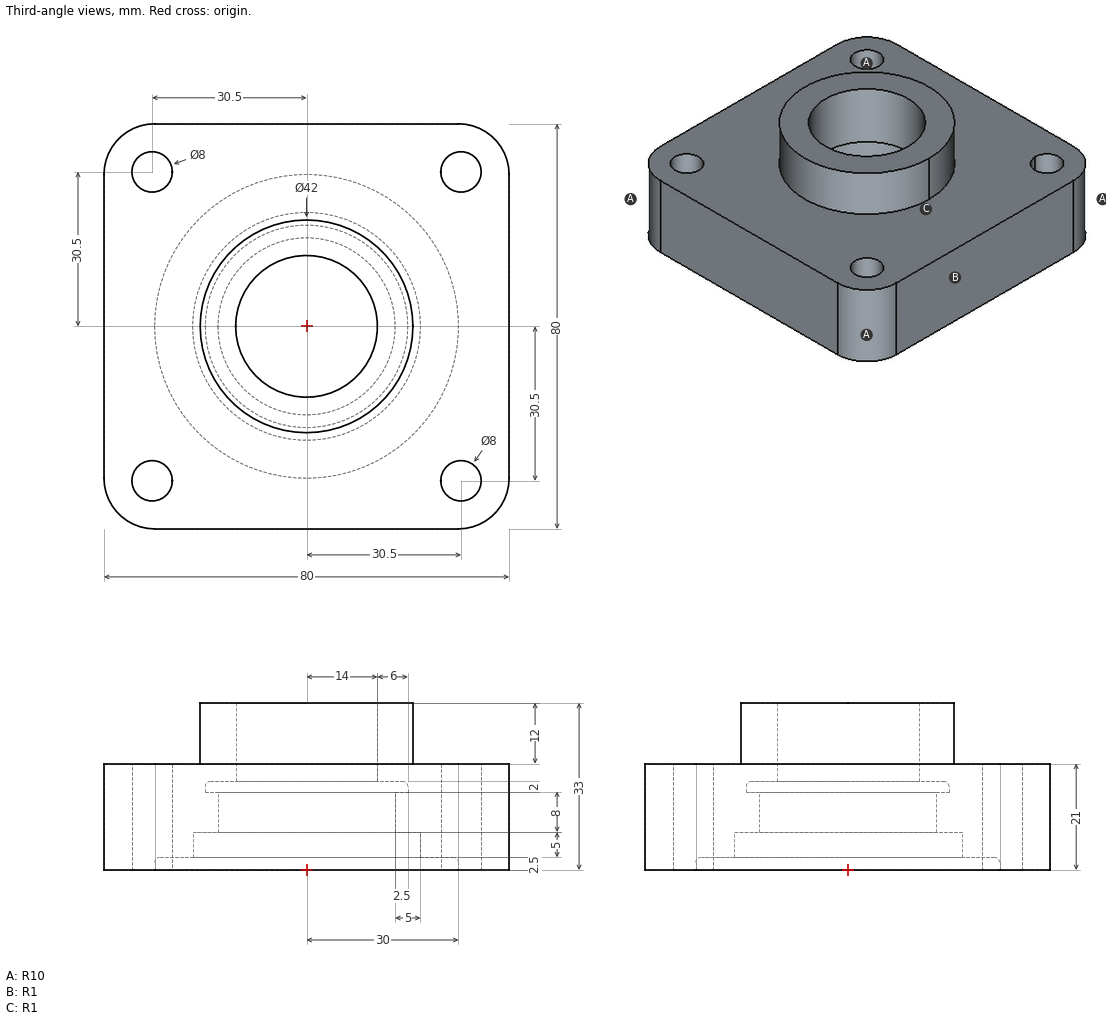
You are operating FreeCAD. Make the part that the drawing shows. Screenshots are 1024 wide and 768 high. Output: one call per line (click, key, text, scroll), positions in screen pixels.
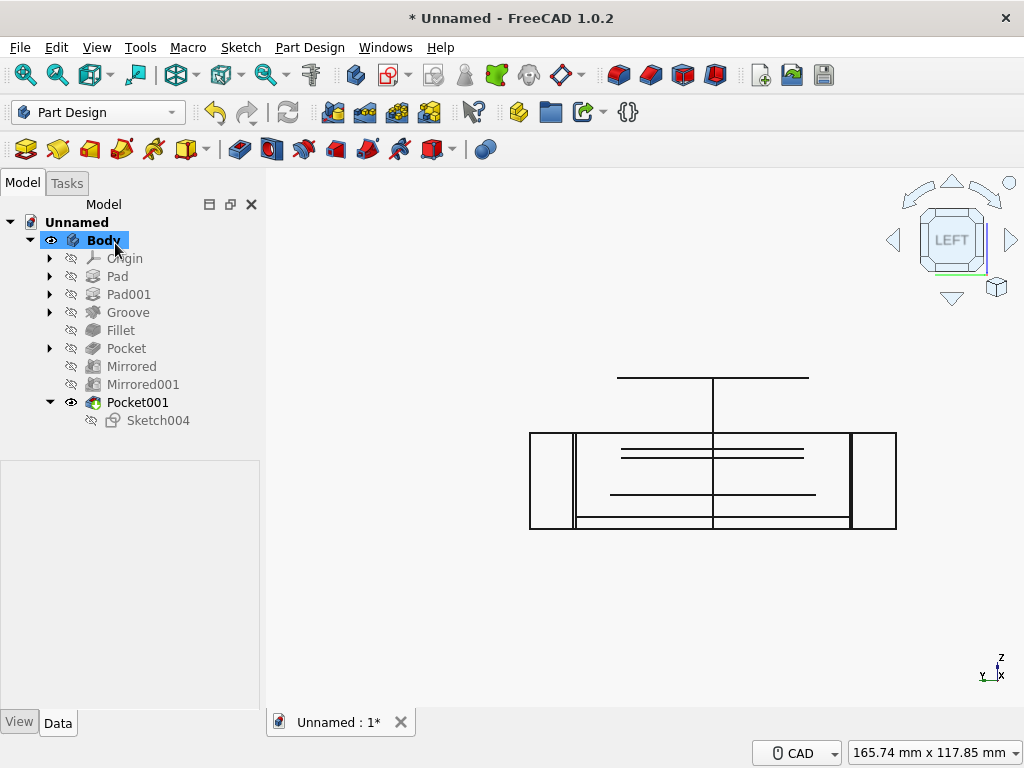
key(0)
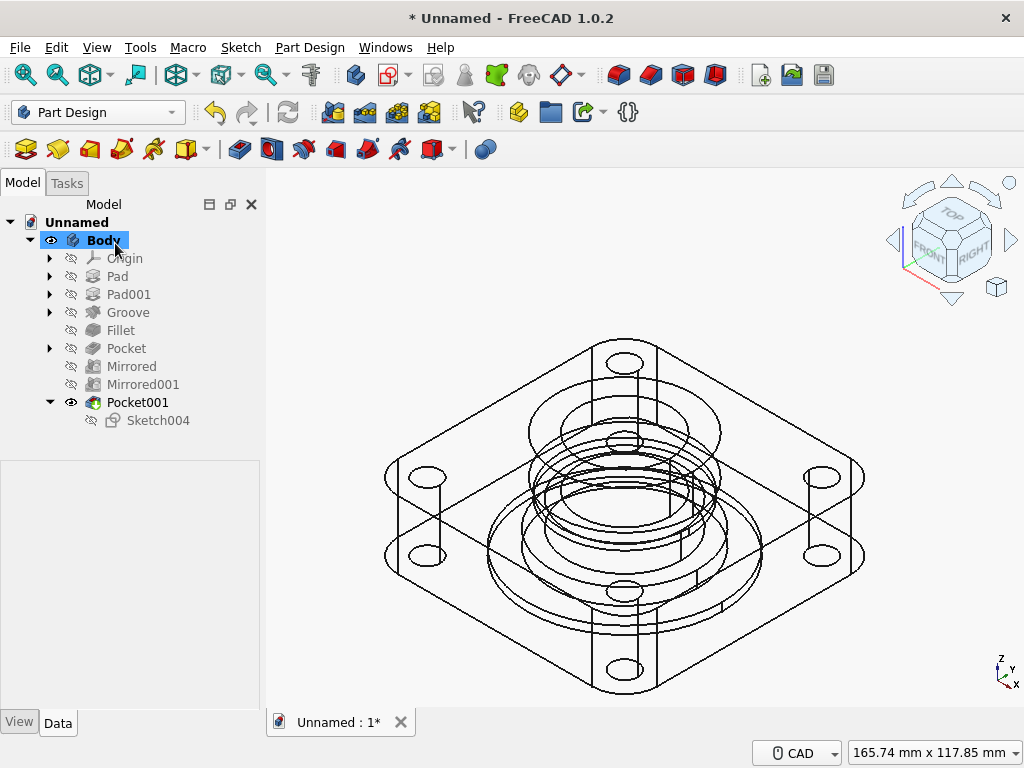
click(489, 533)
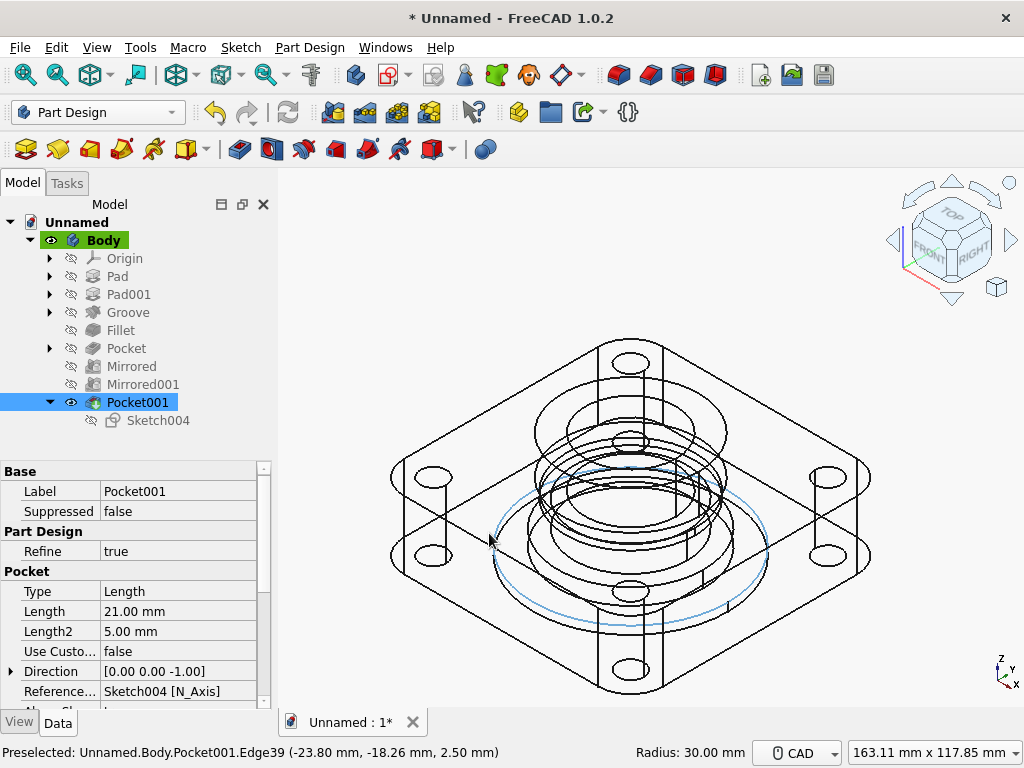
key(v)
key(1)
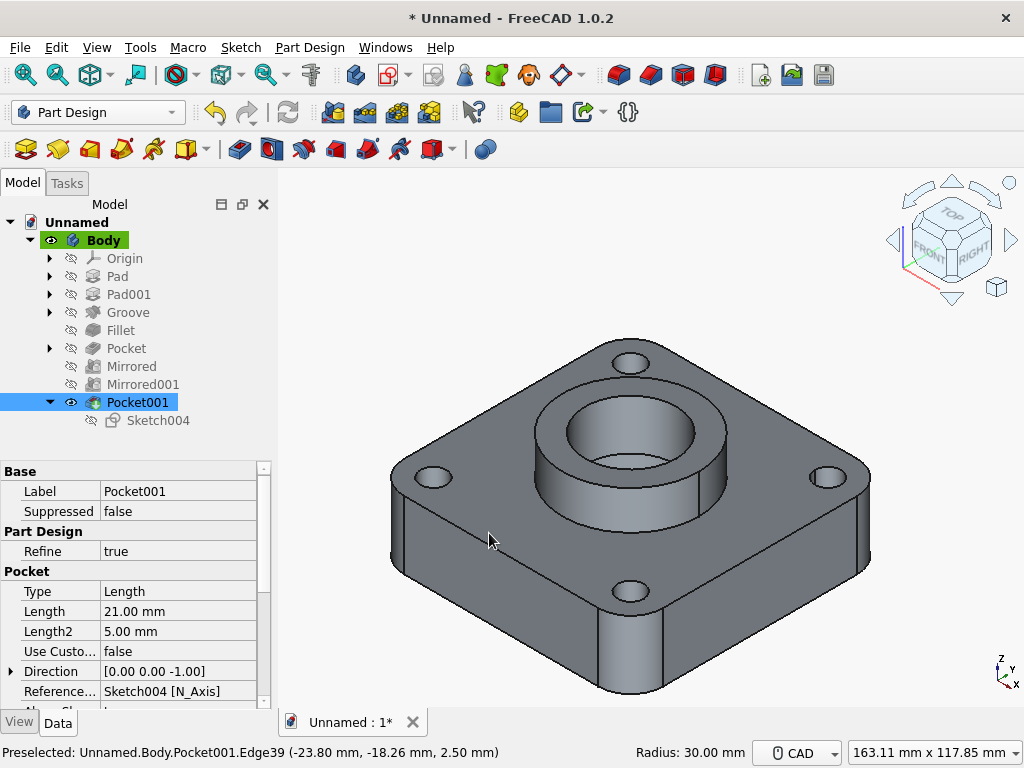
click(620, 76)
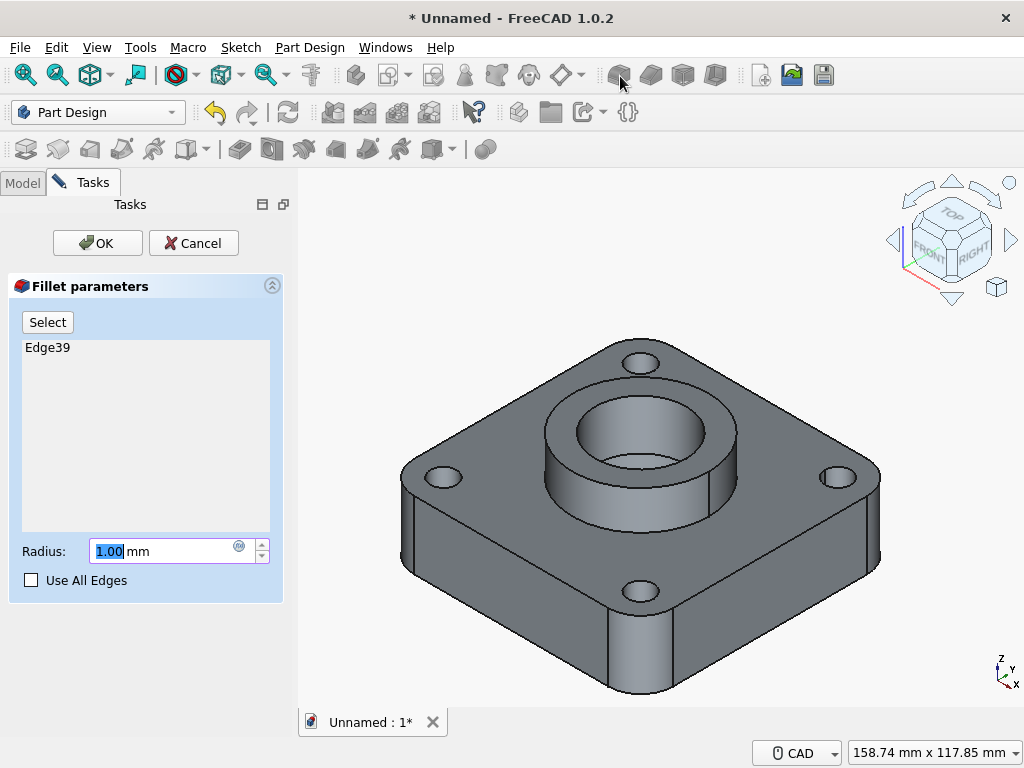
text(1)
key(Tab)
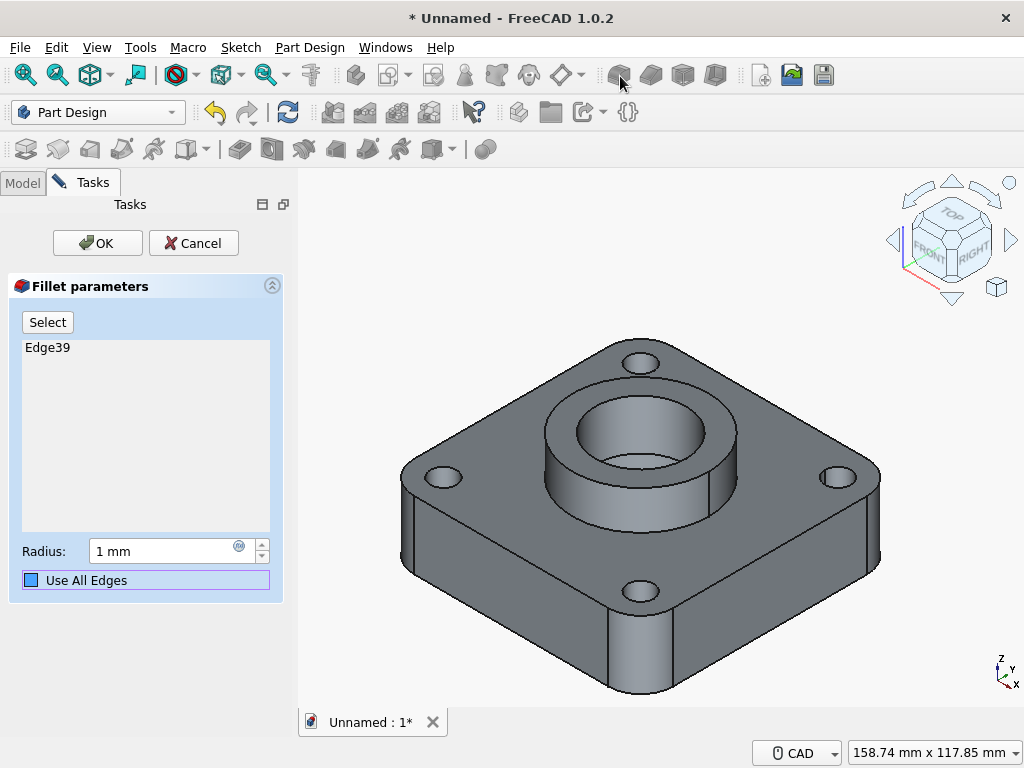
click(98, 243)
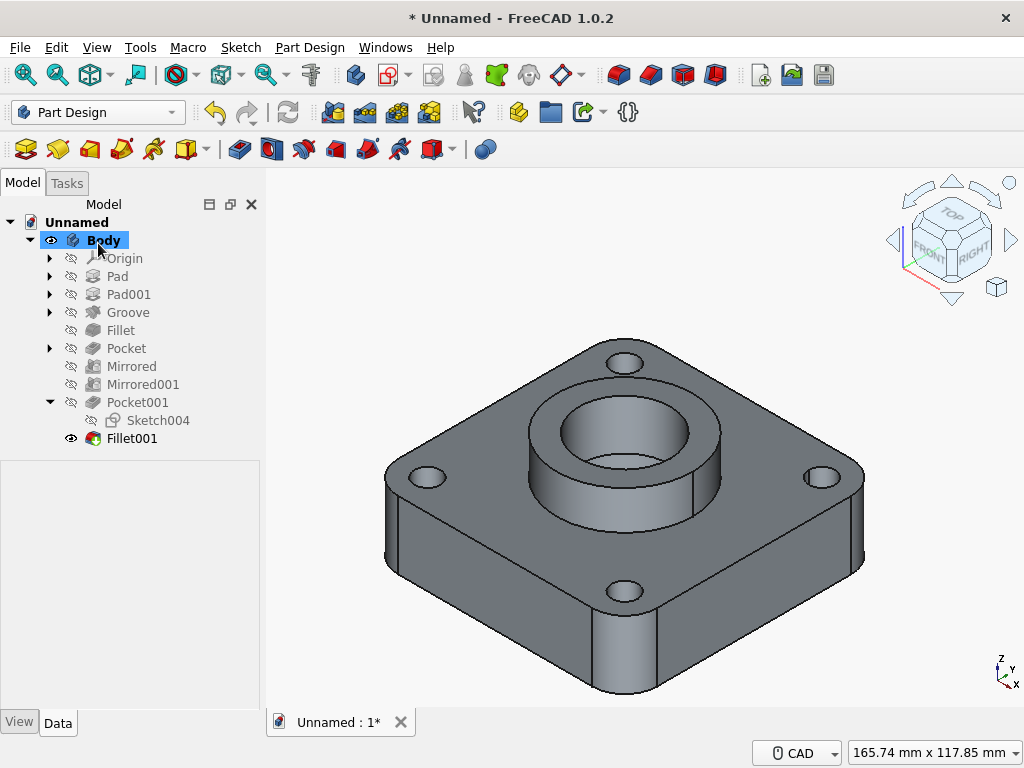
key(2)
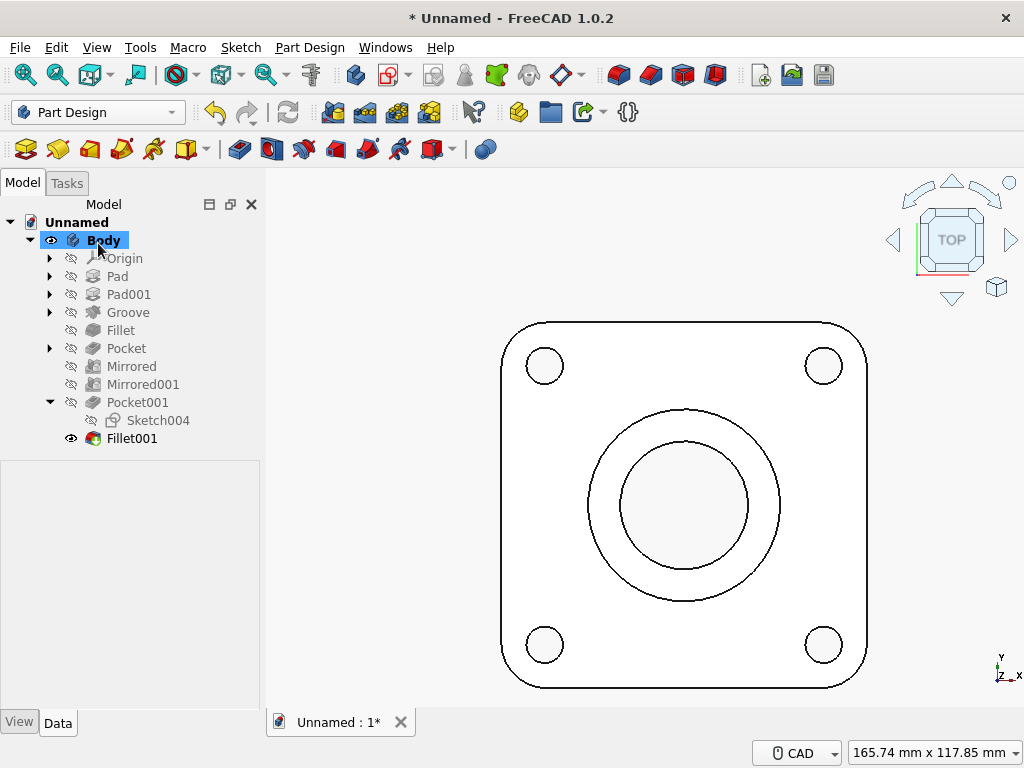
key(0)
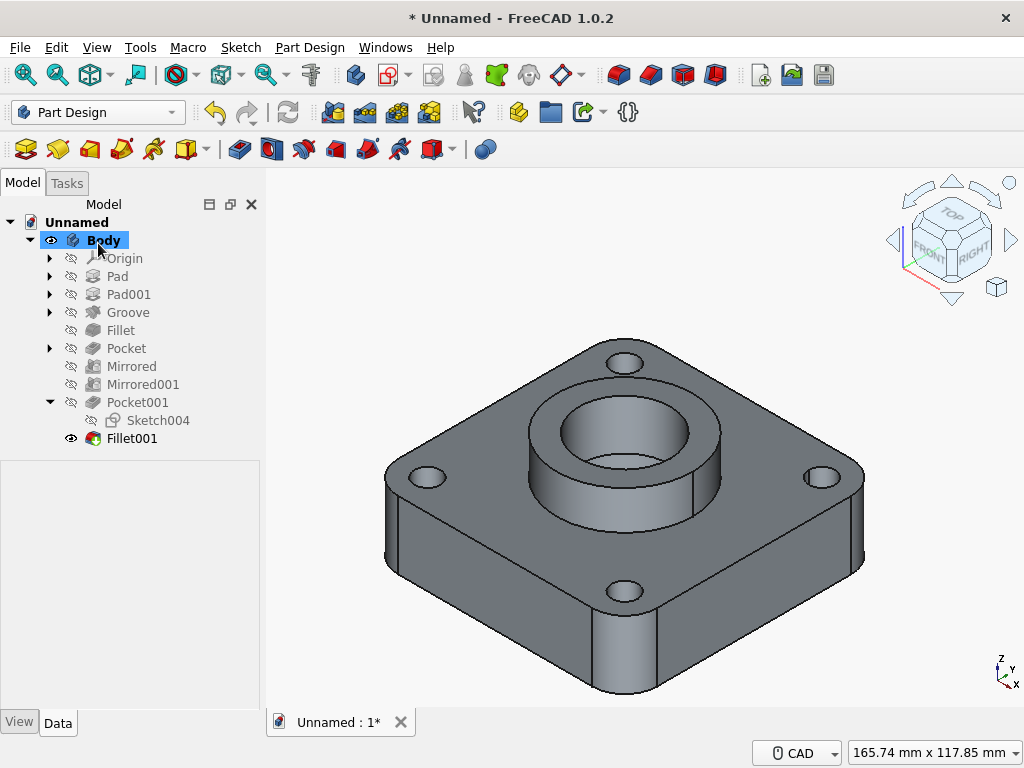
key(1)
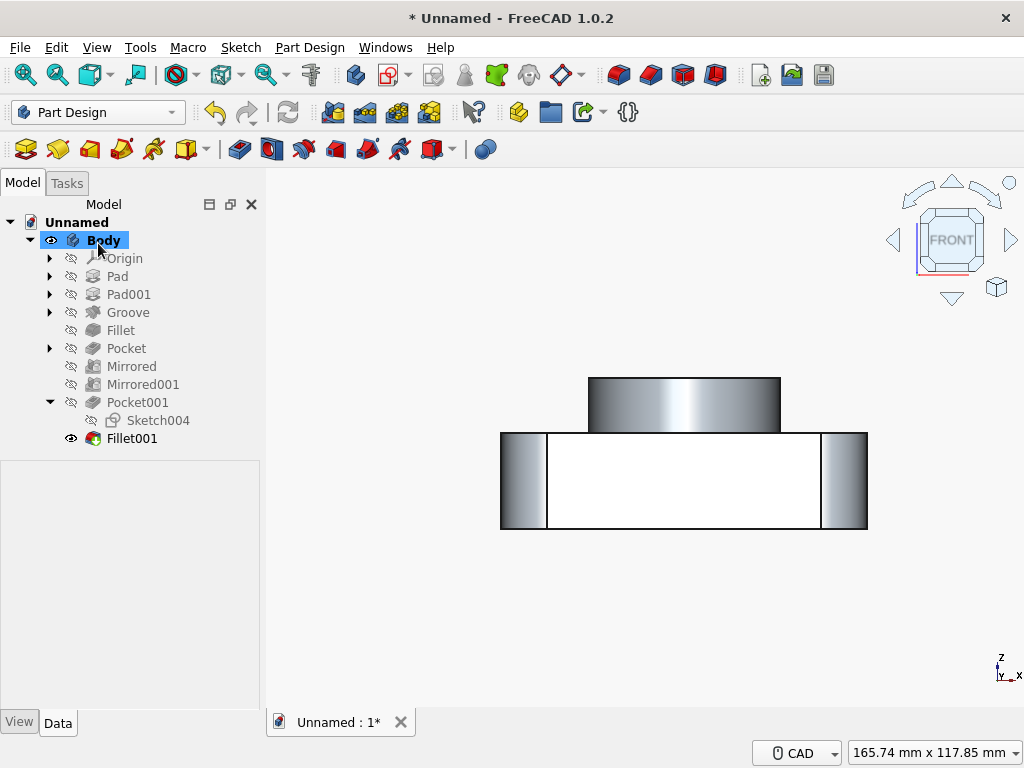
key(3)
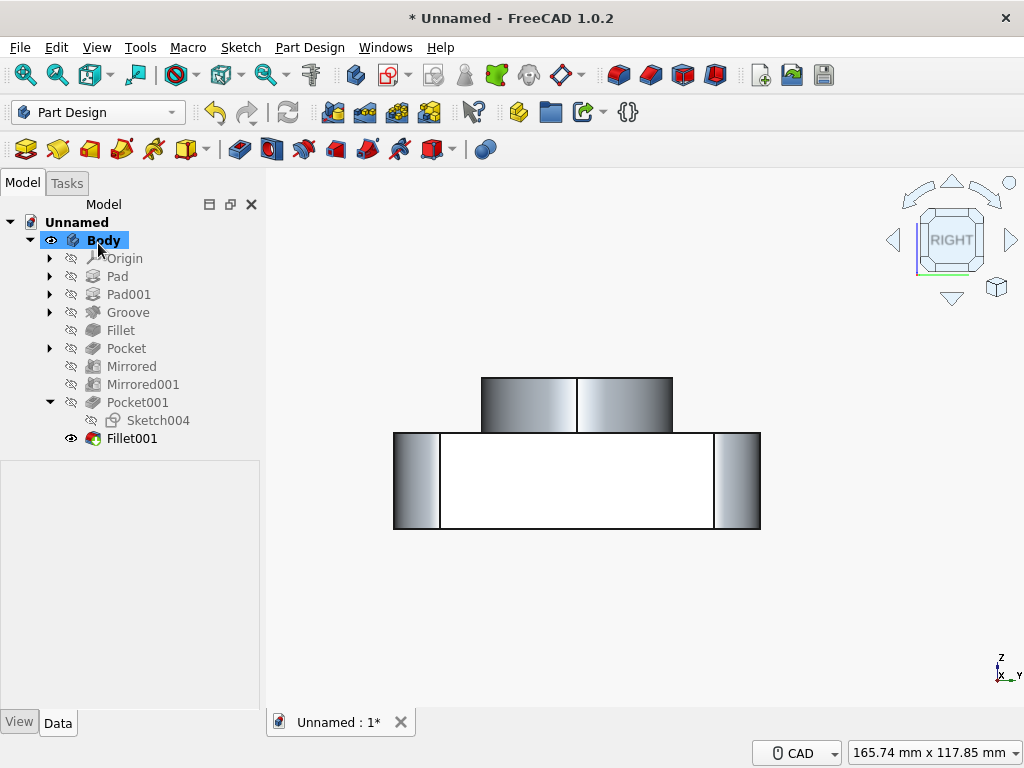
key(5)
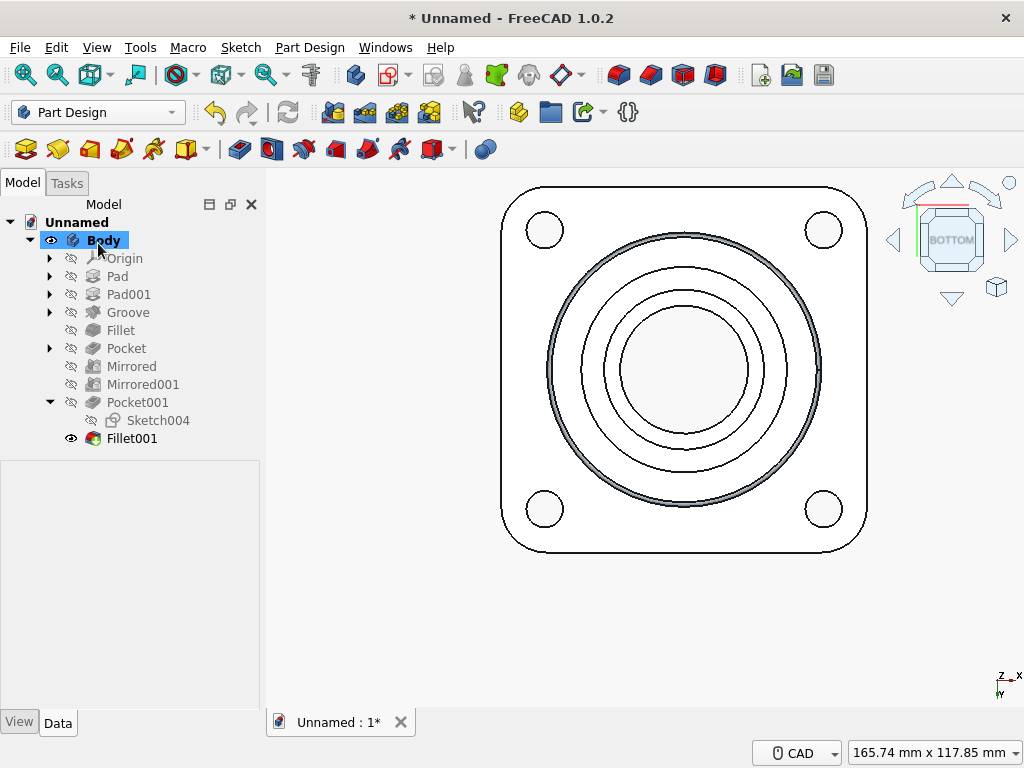
key(4)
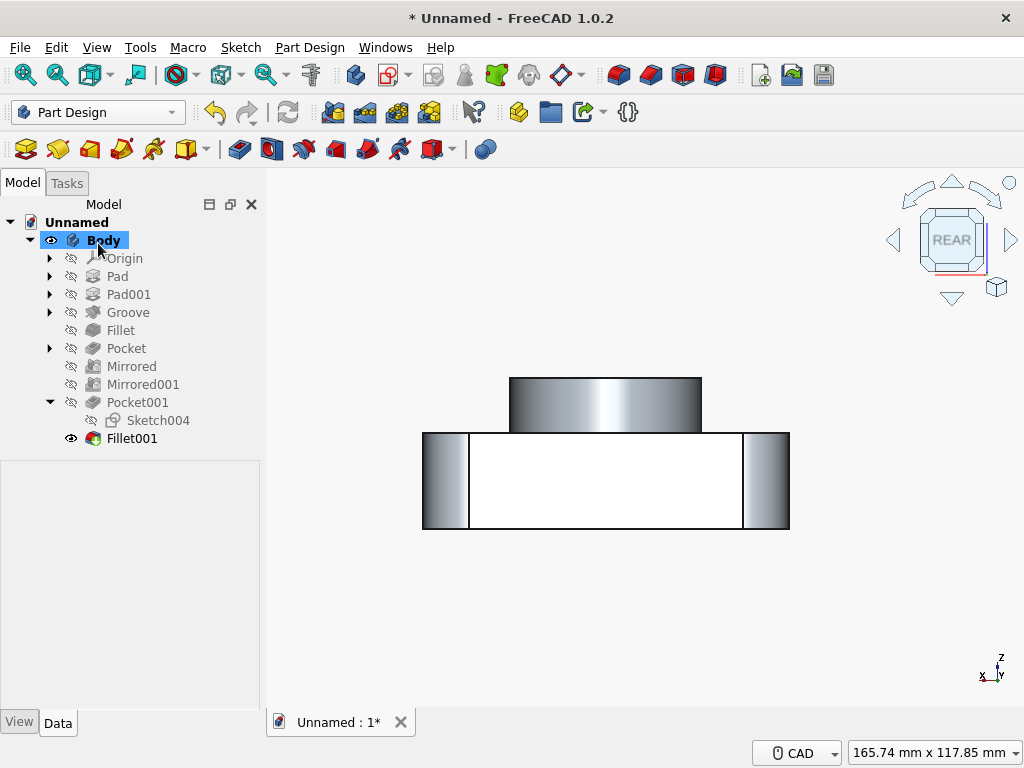
key(6)